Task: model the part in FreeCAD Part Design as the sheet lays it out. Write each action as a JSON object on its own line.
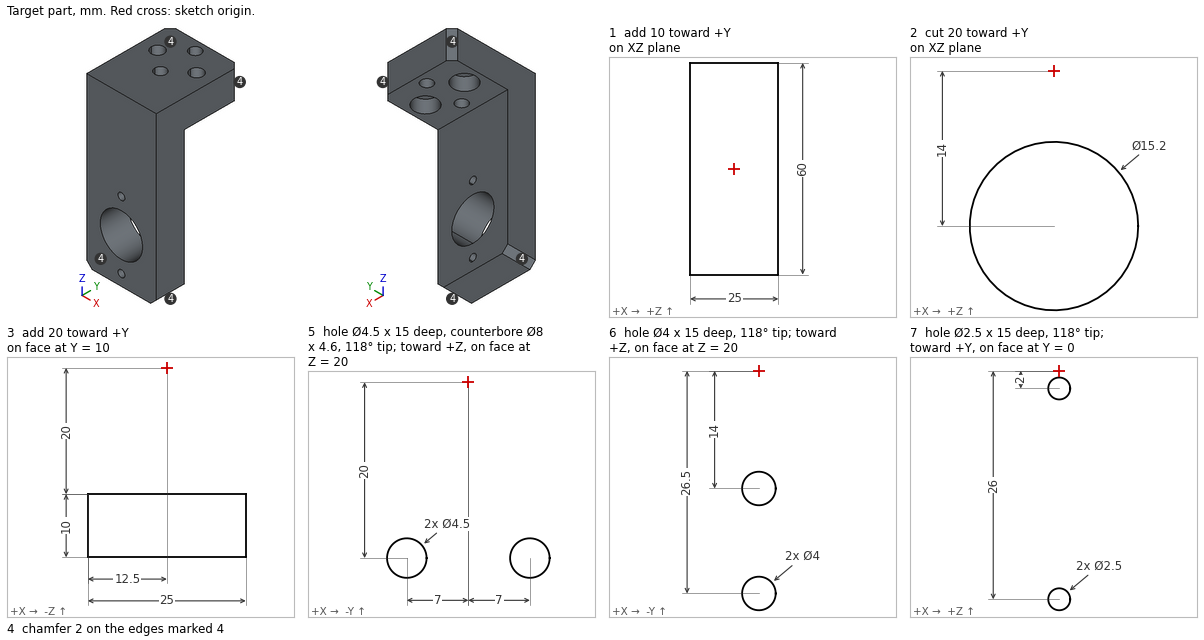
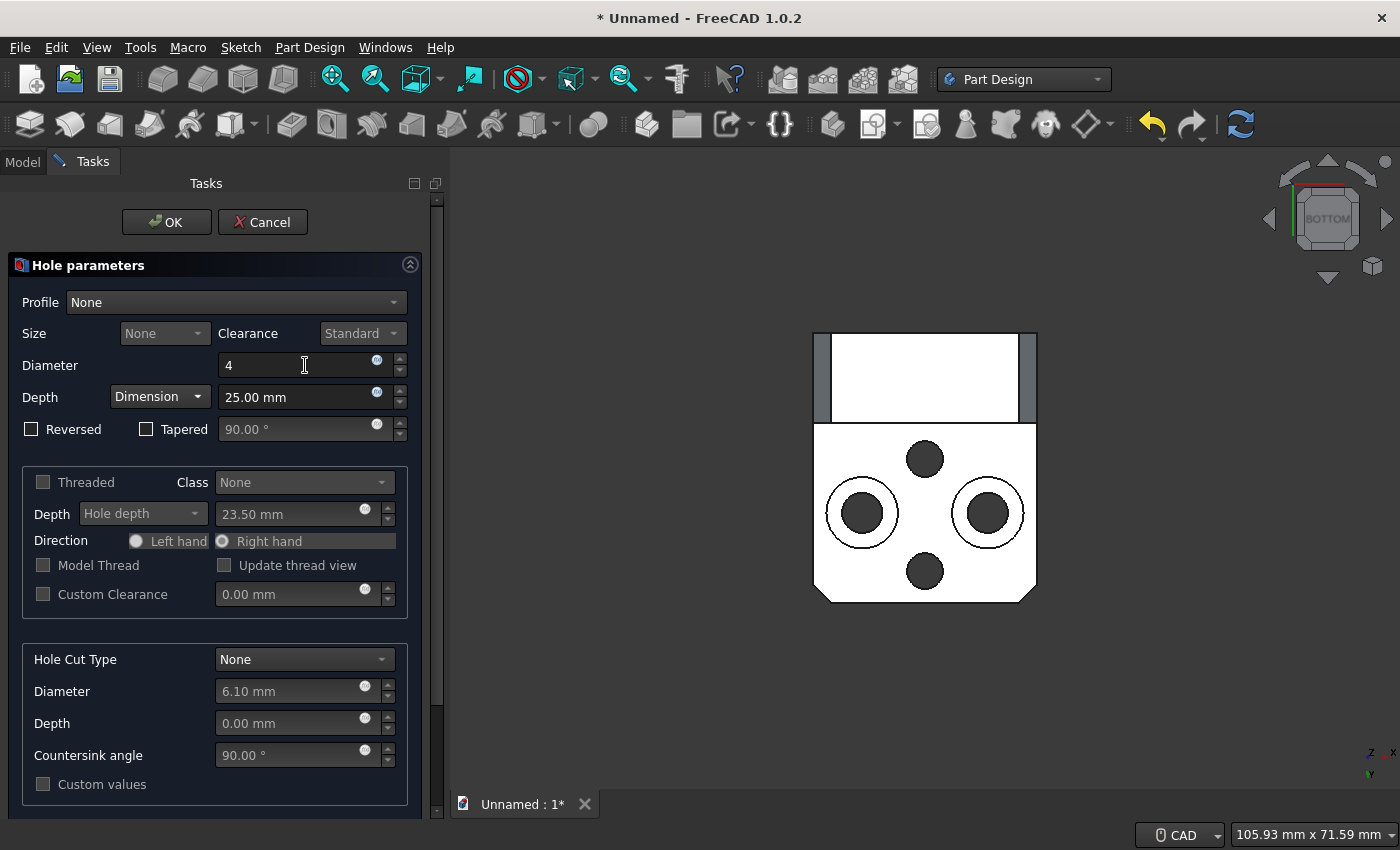
{"action": "triple_click", "coordinate": [305, 397]}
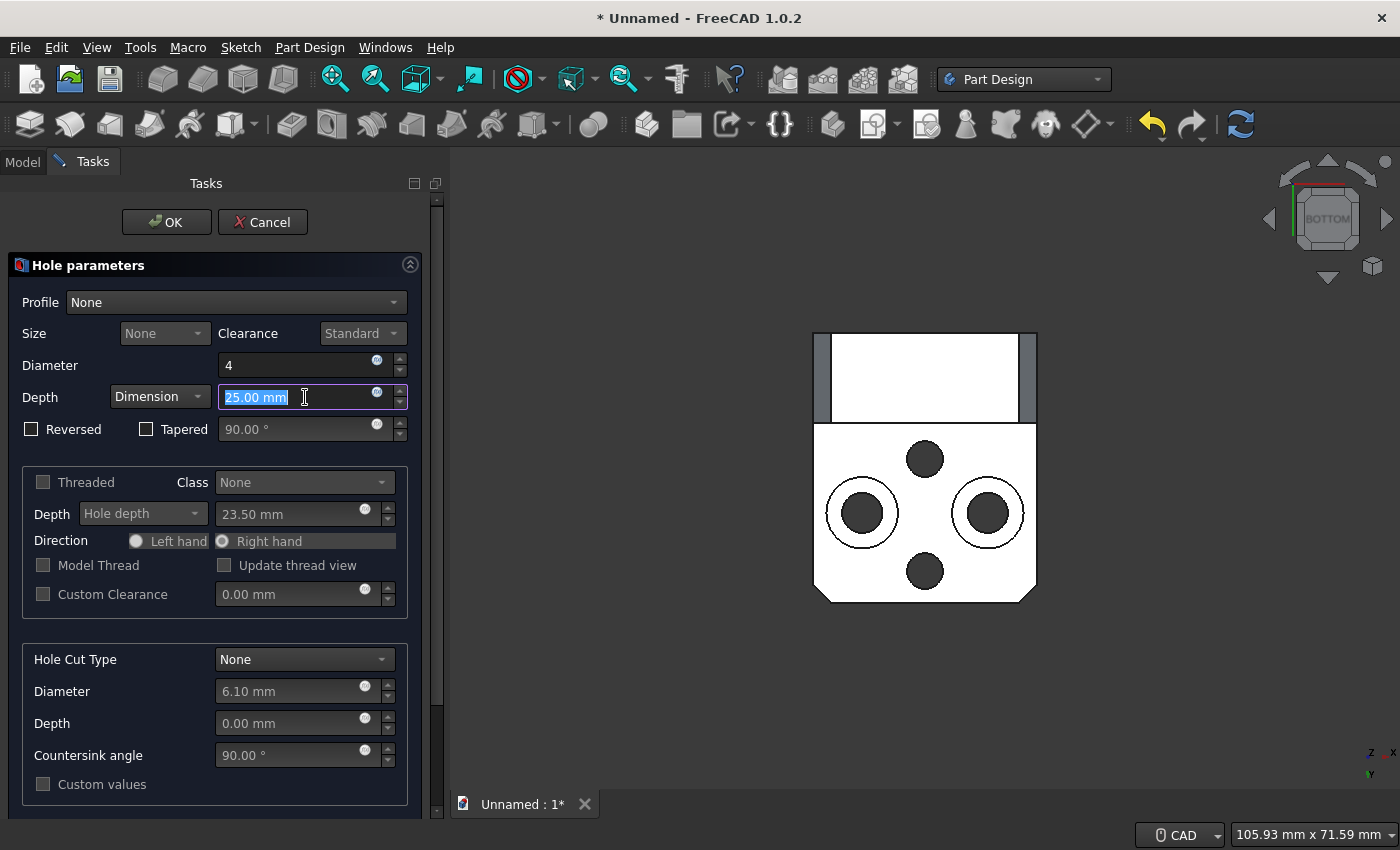
{"action": "type", "text": "15"}
{"action": "key", "text": "Tab"}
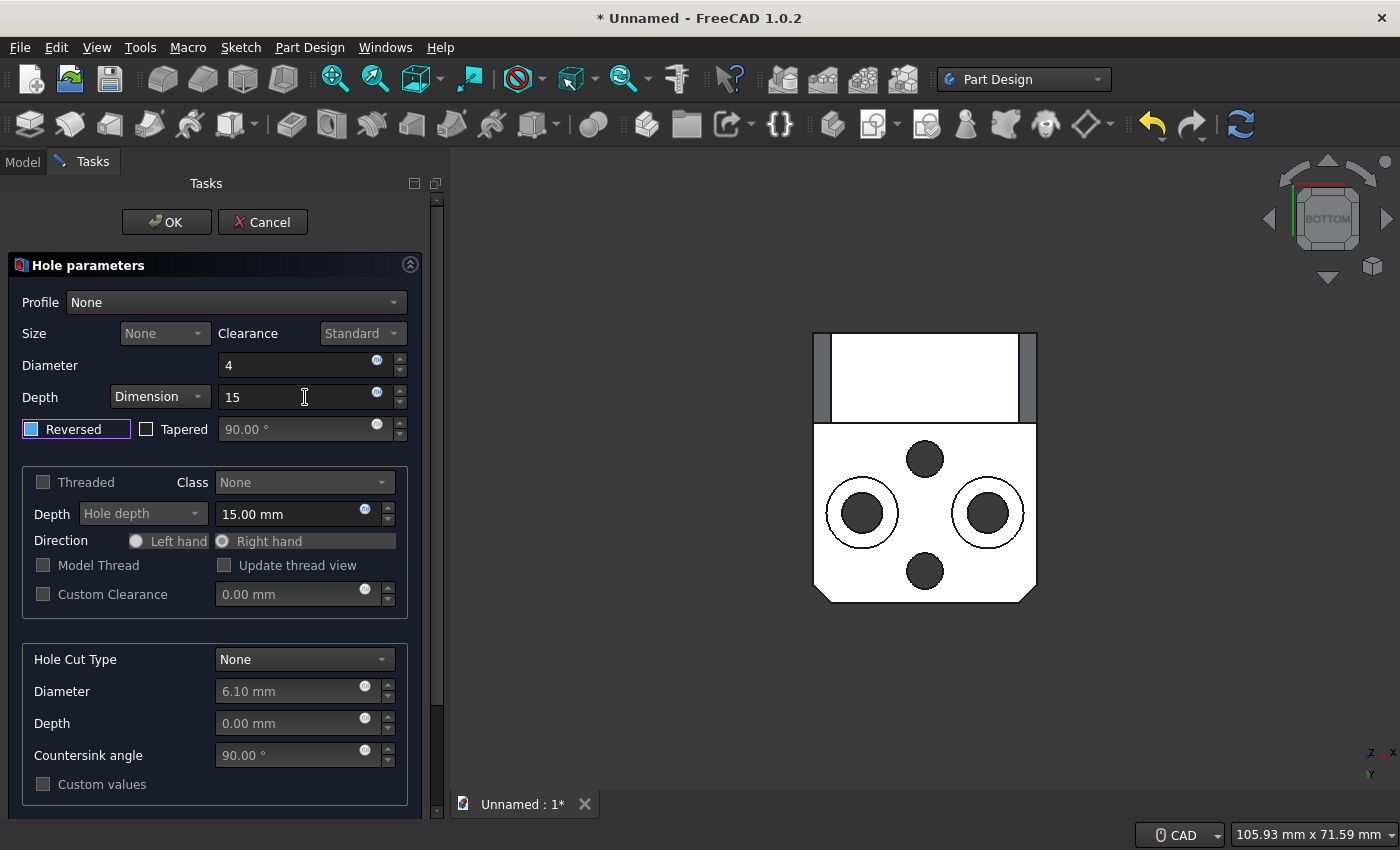
{"action": "left_click", "coordinate": [167, 222]}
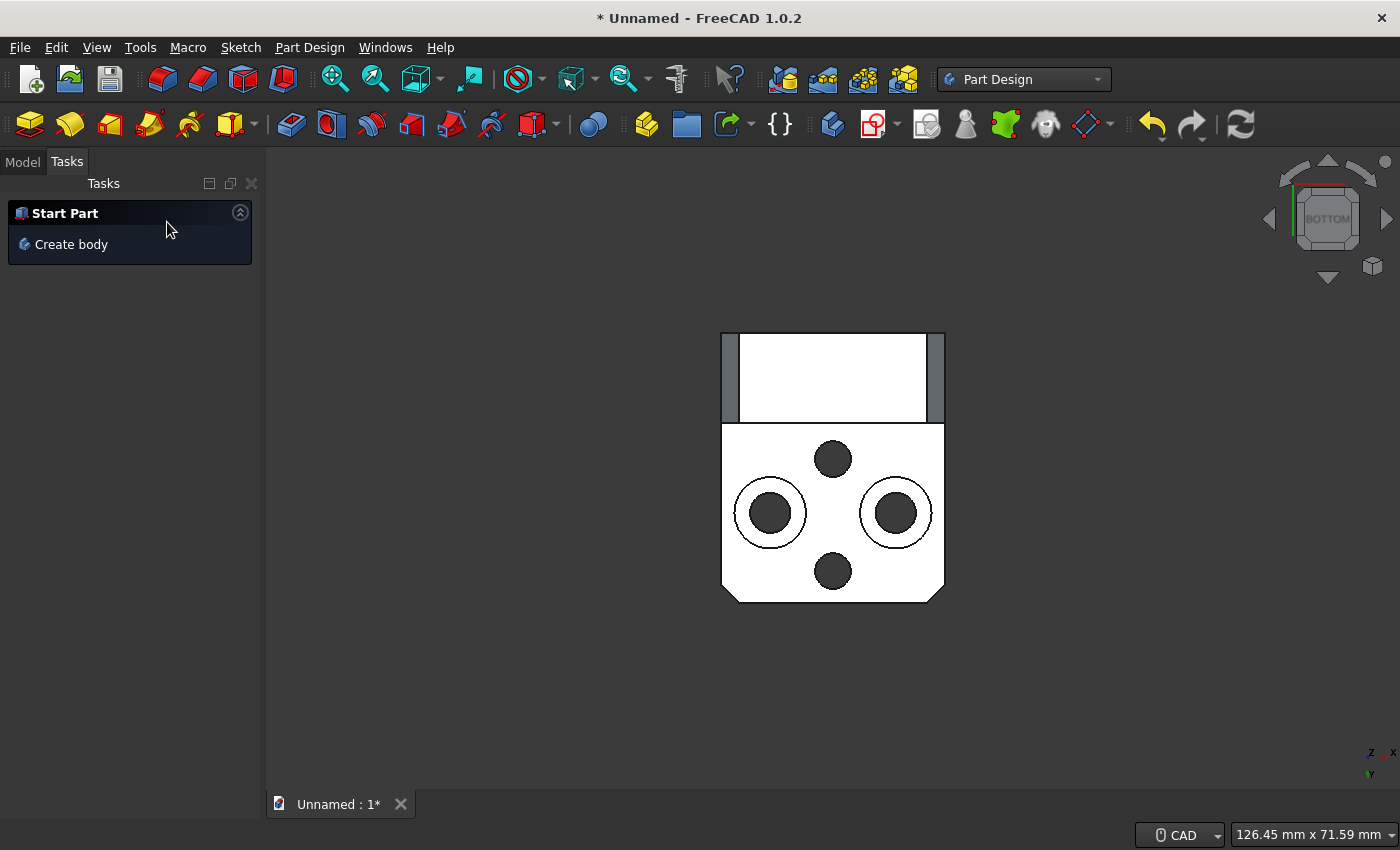
{"action": "left_click", "coordinate": [336, 80]}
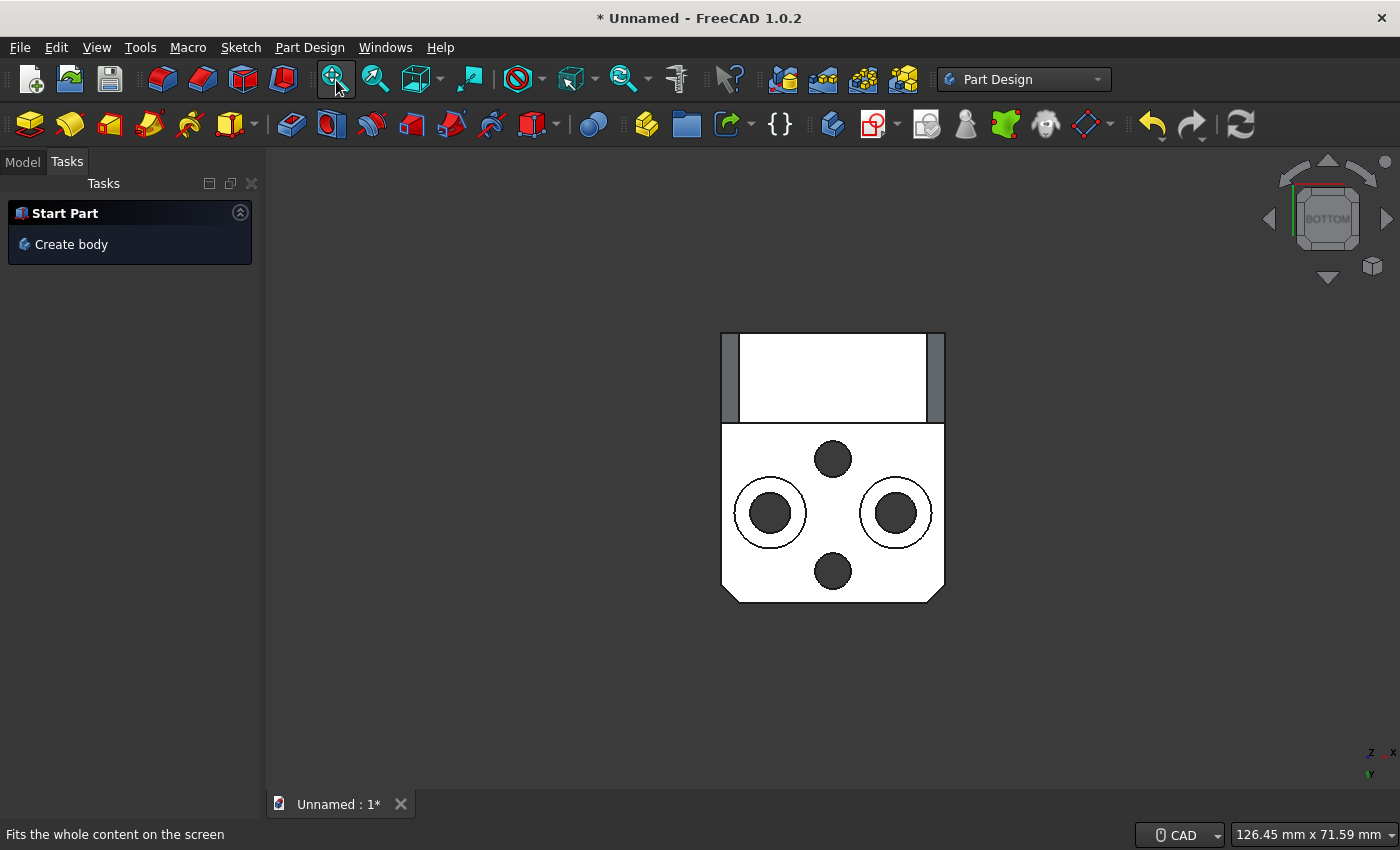
{"action": "key", "text": "0"}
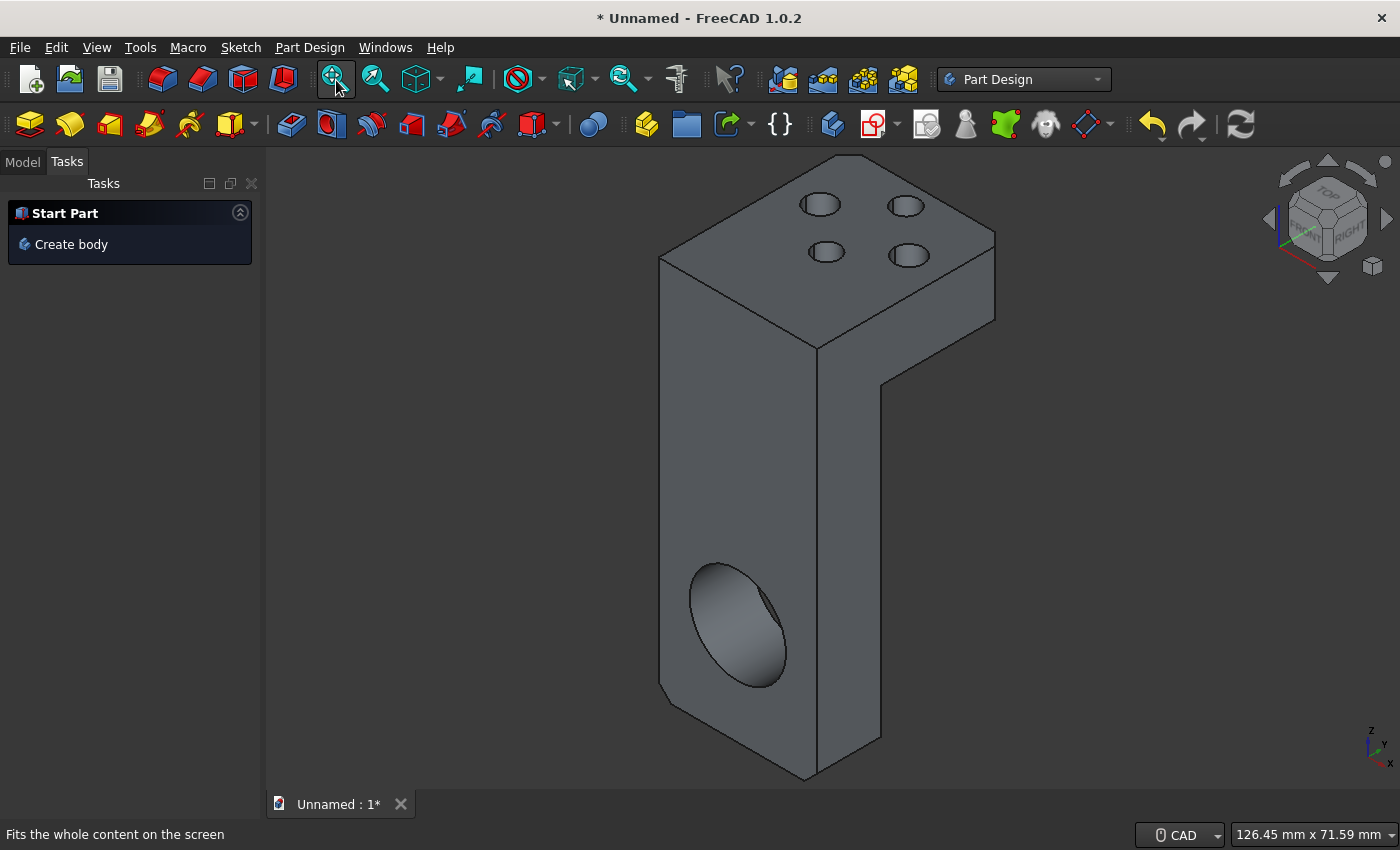
{"action": "left_click", "coordinate": [738, 396]}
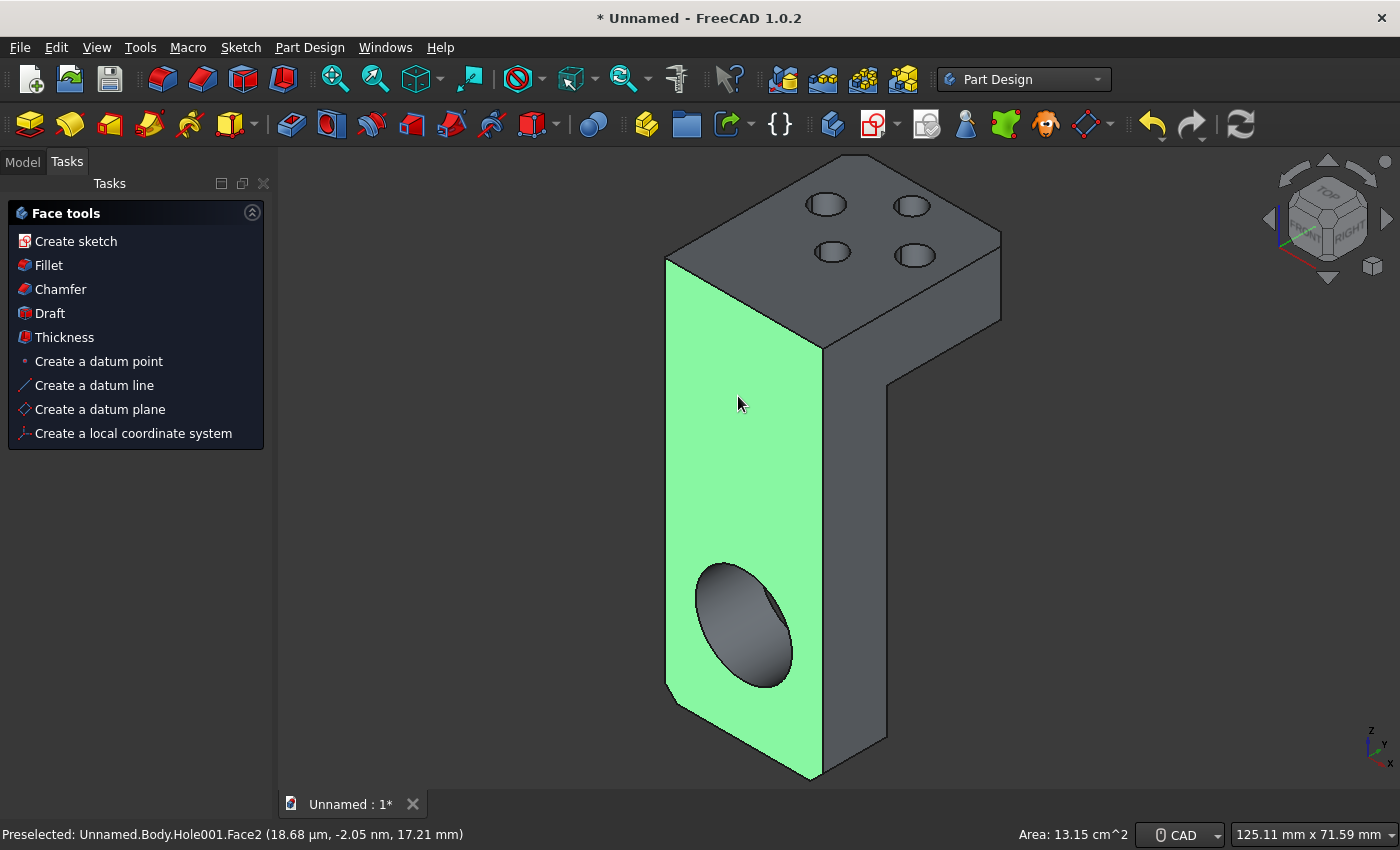
{"action": "left_click", "coordinate": [874, 124]}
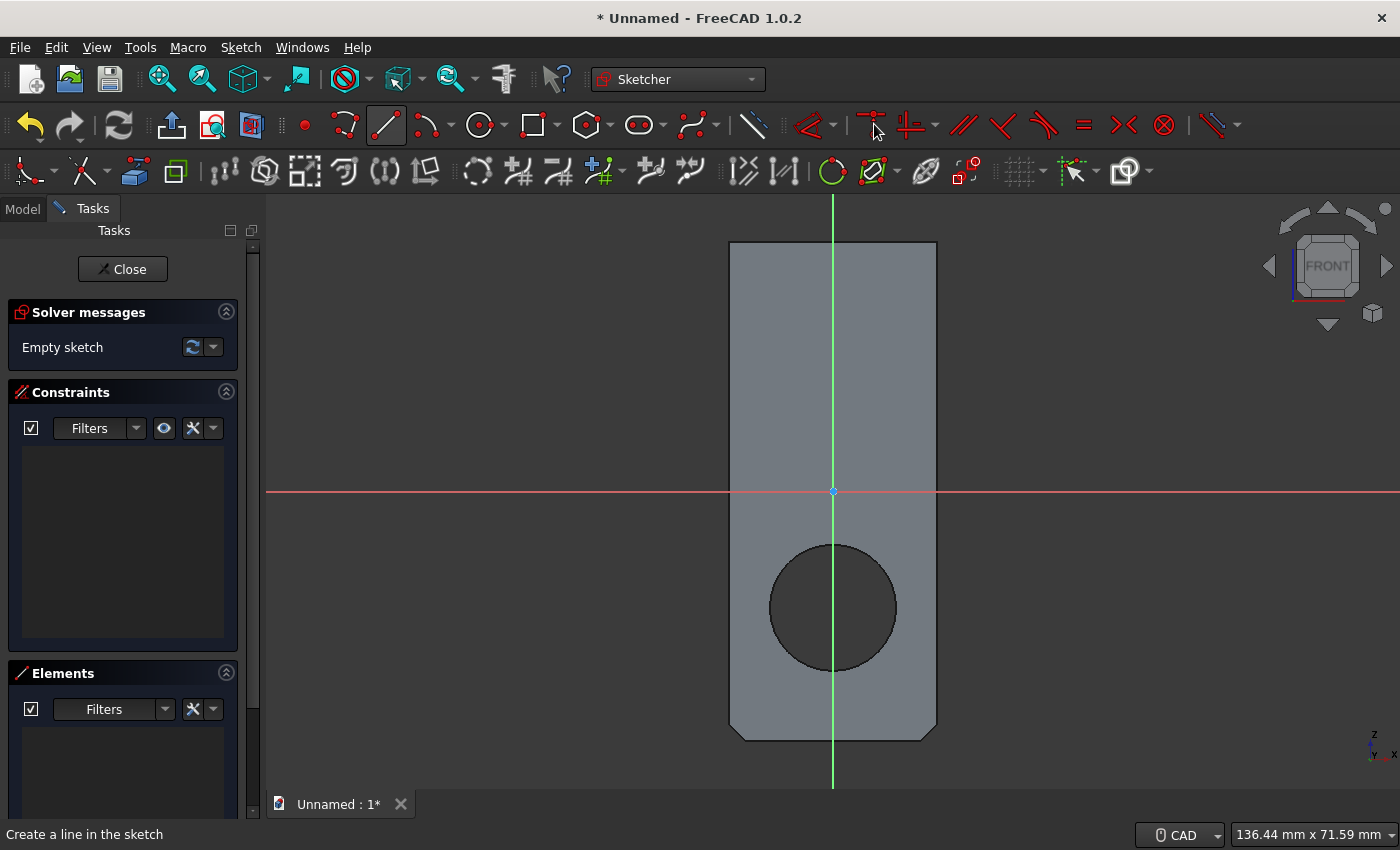
{"action": "scroll", "coordinate": [916, 742], "scroll_direction": "up", "scroll_amount": 3}